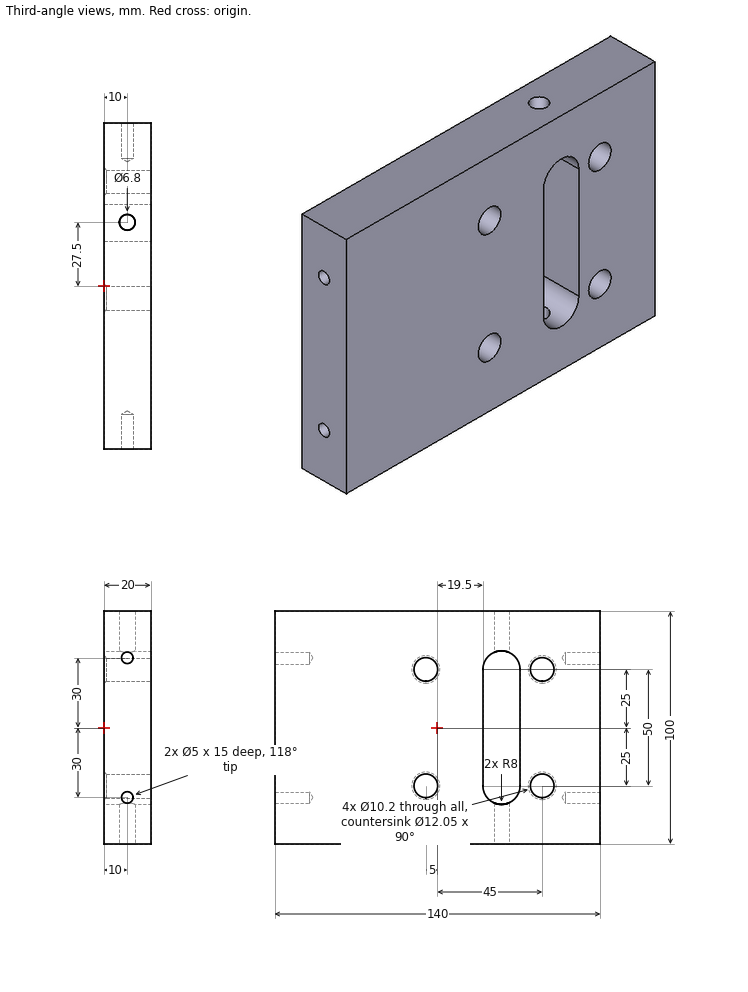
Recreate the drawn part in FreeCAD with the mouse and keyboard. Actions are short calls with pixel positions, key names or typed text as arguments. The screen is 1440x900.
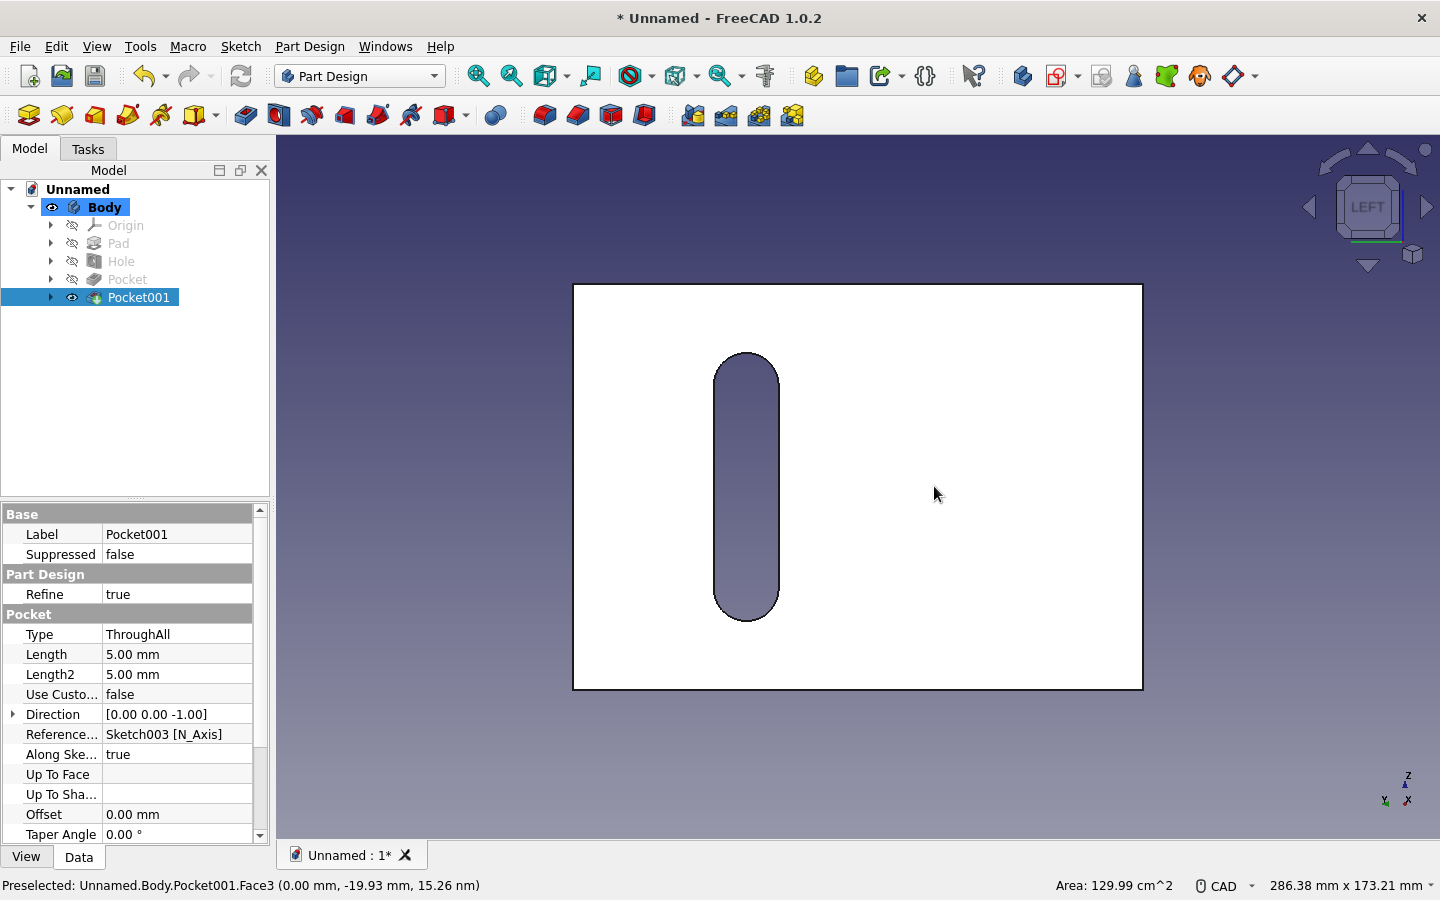
click(1056, 76)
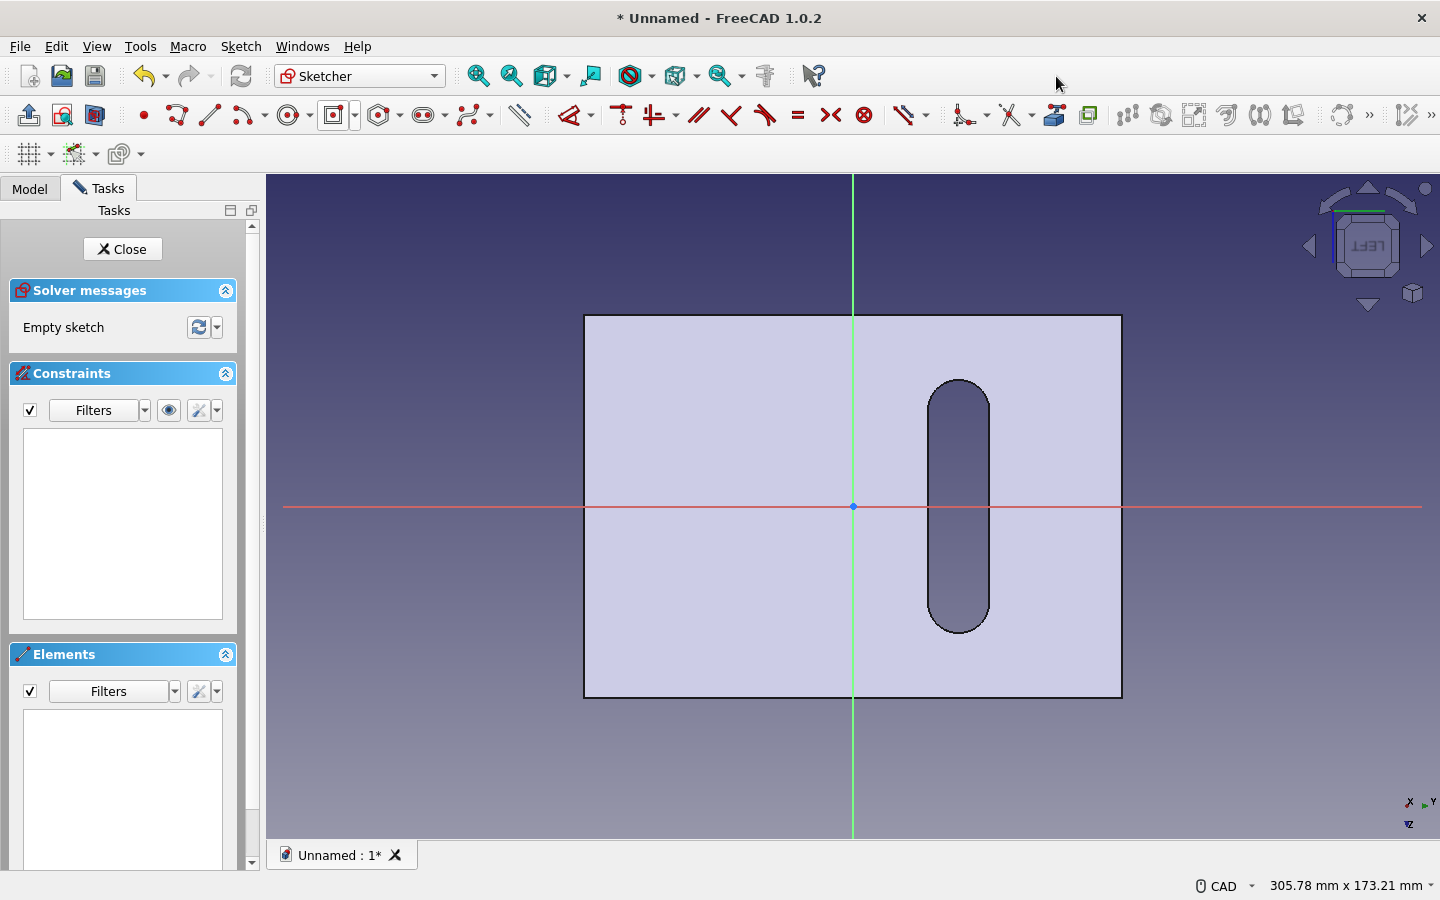
scroll(1107, 506, up, 3)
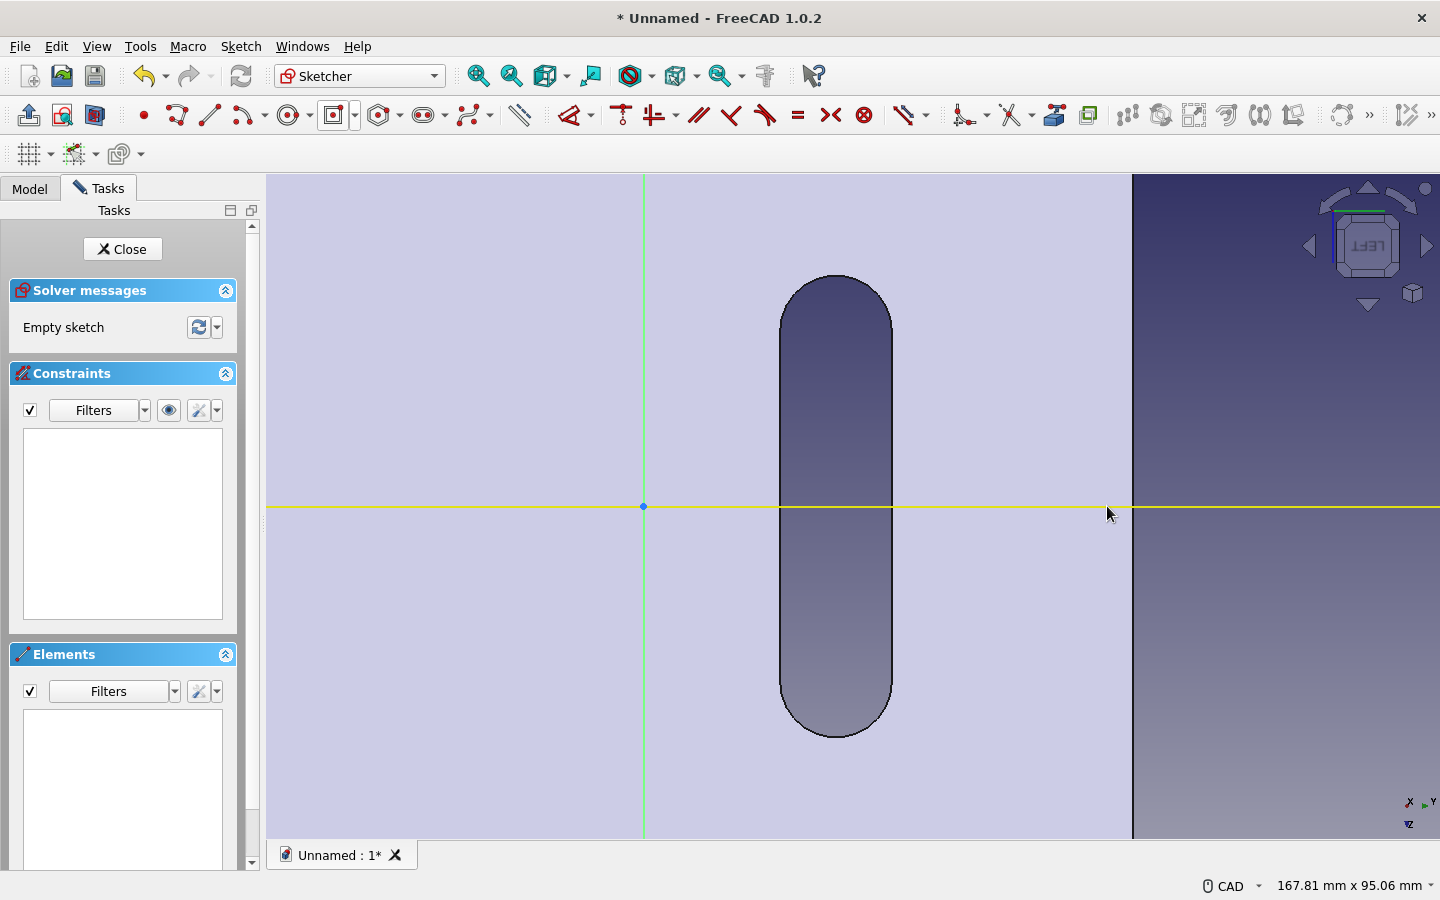
click(288, 116)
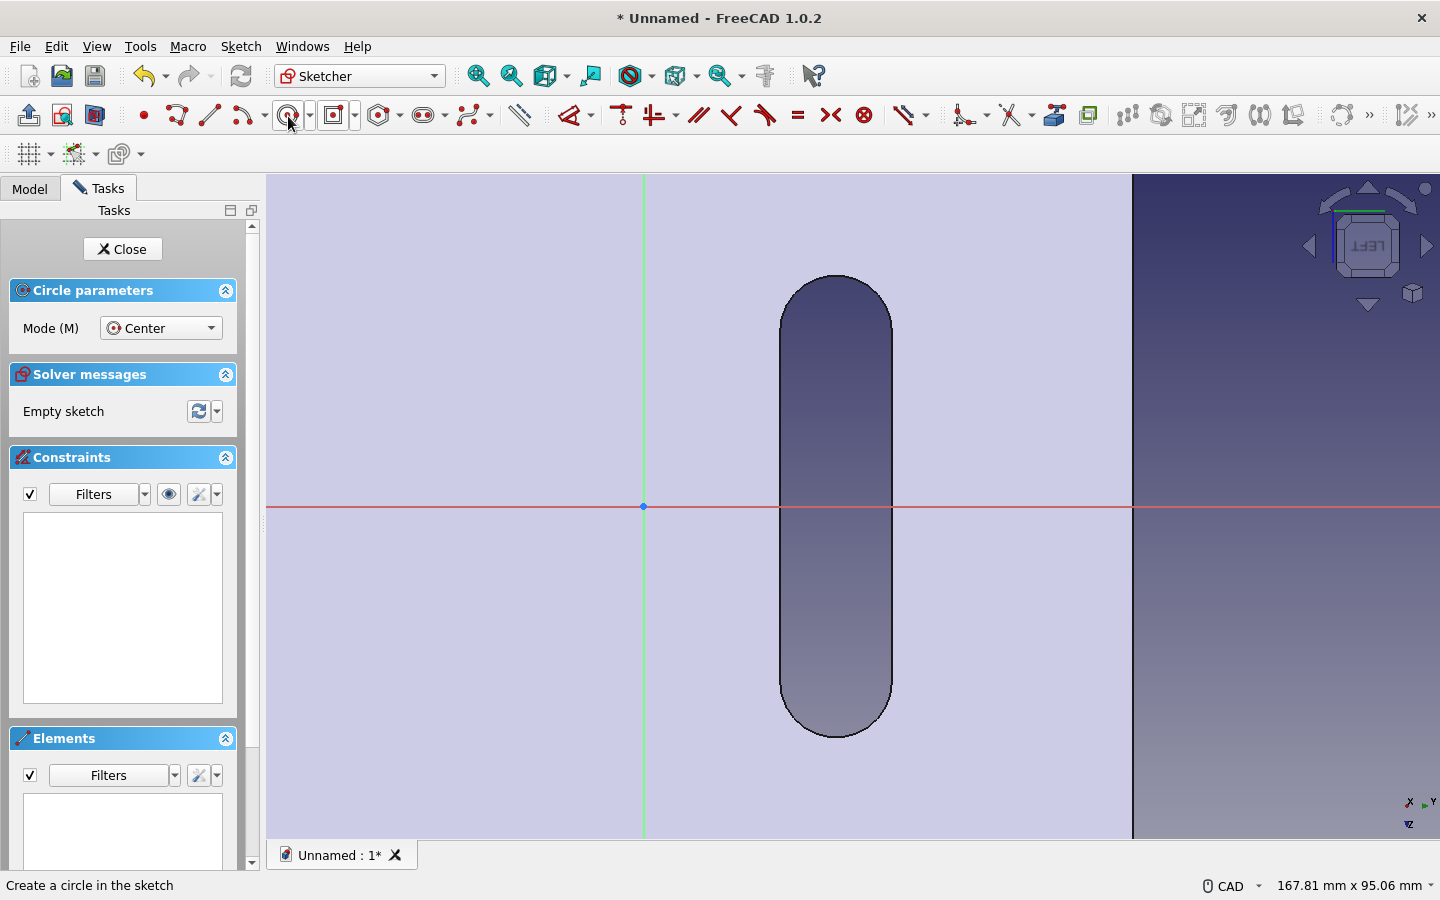
click(958, 332)
move(984, 306)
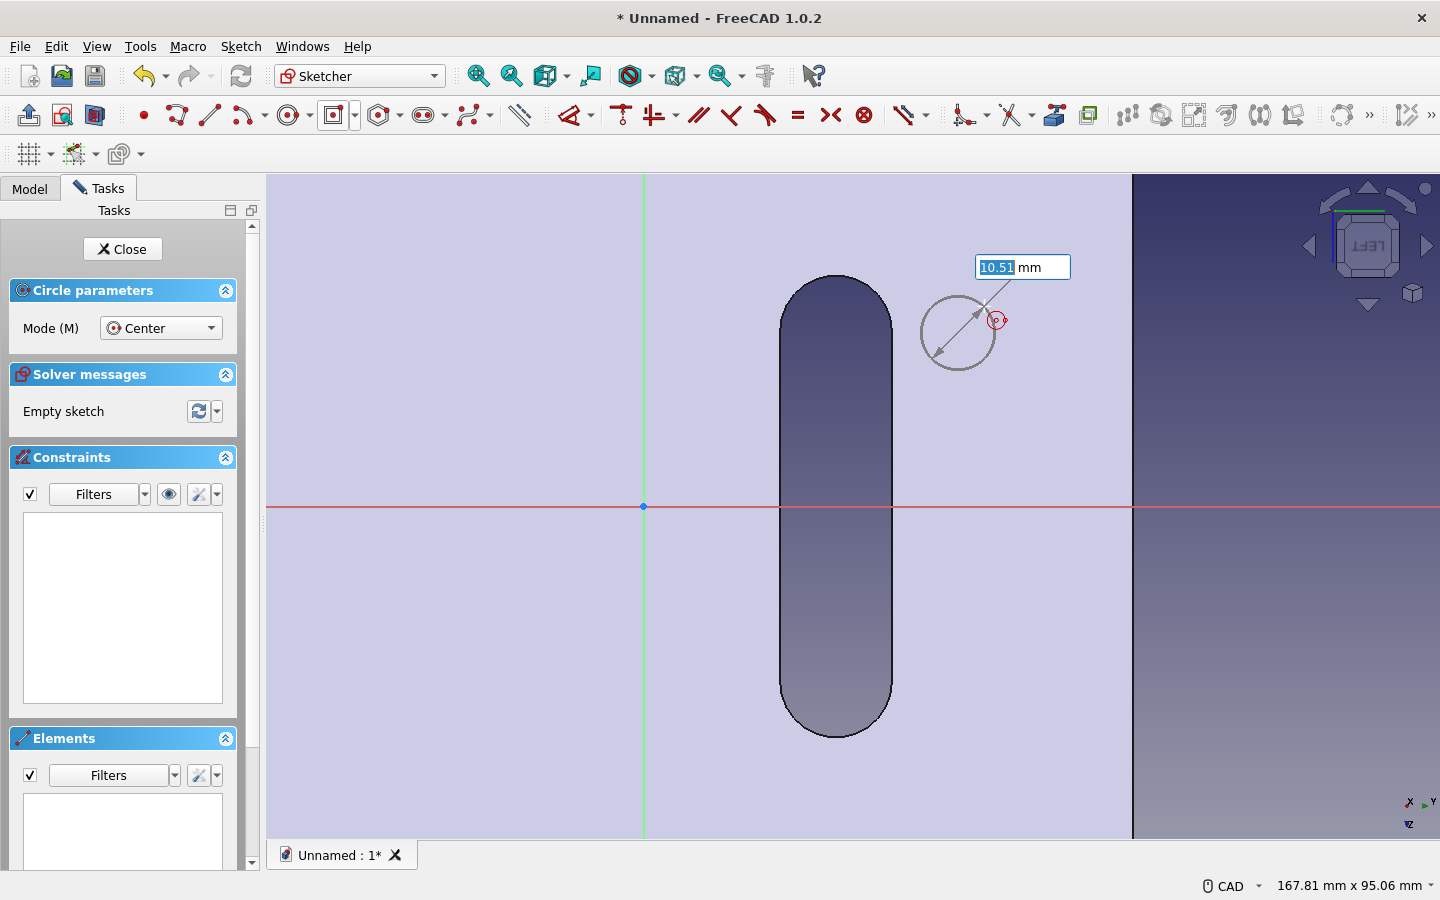
text(10.2)
key(Return)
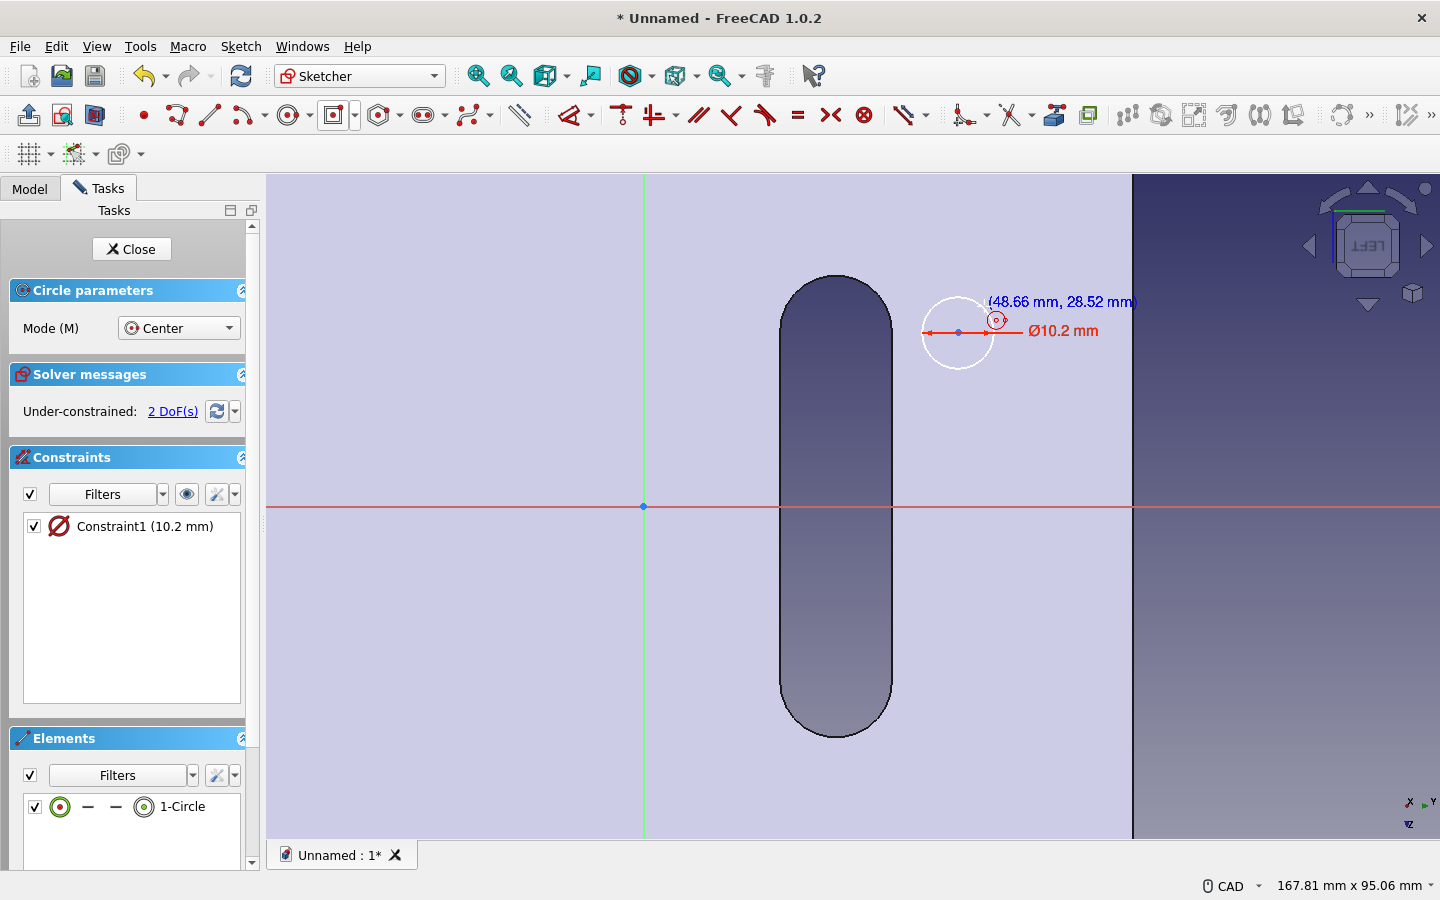
click(958, 681)
move(984, 656)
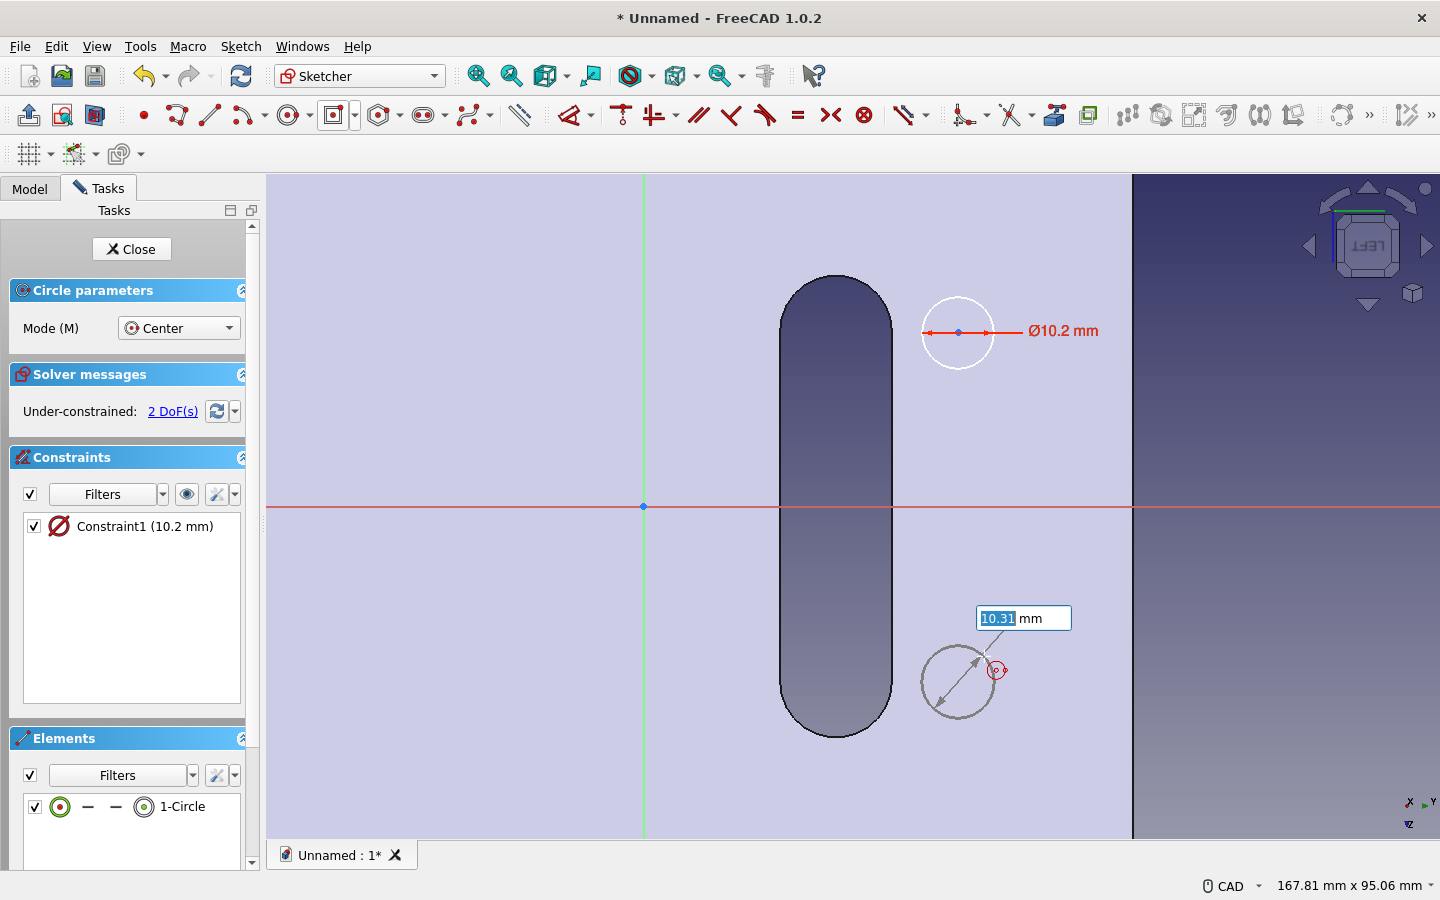
text(10.2)
key(Return)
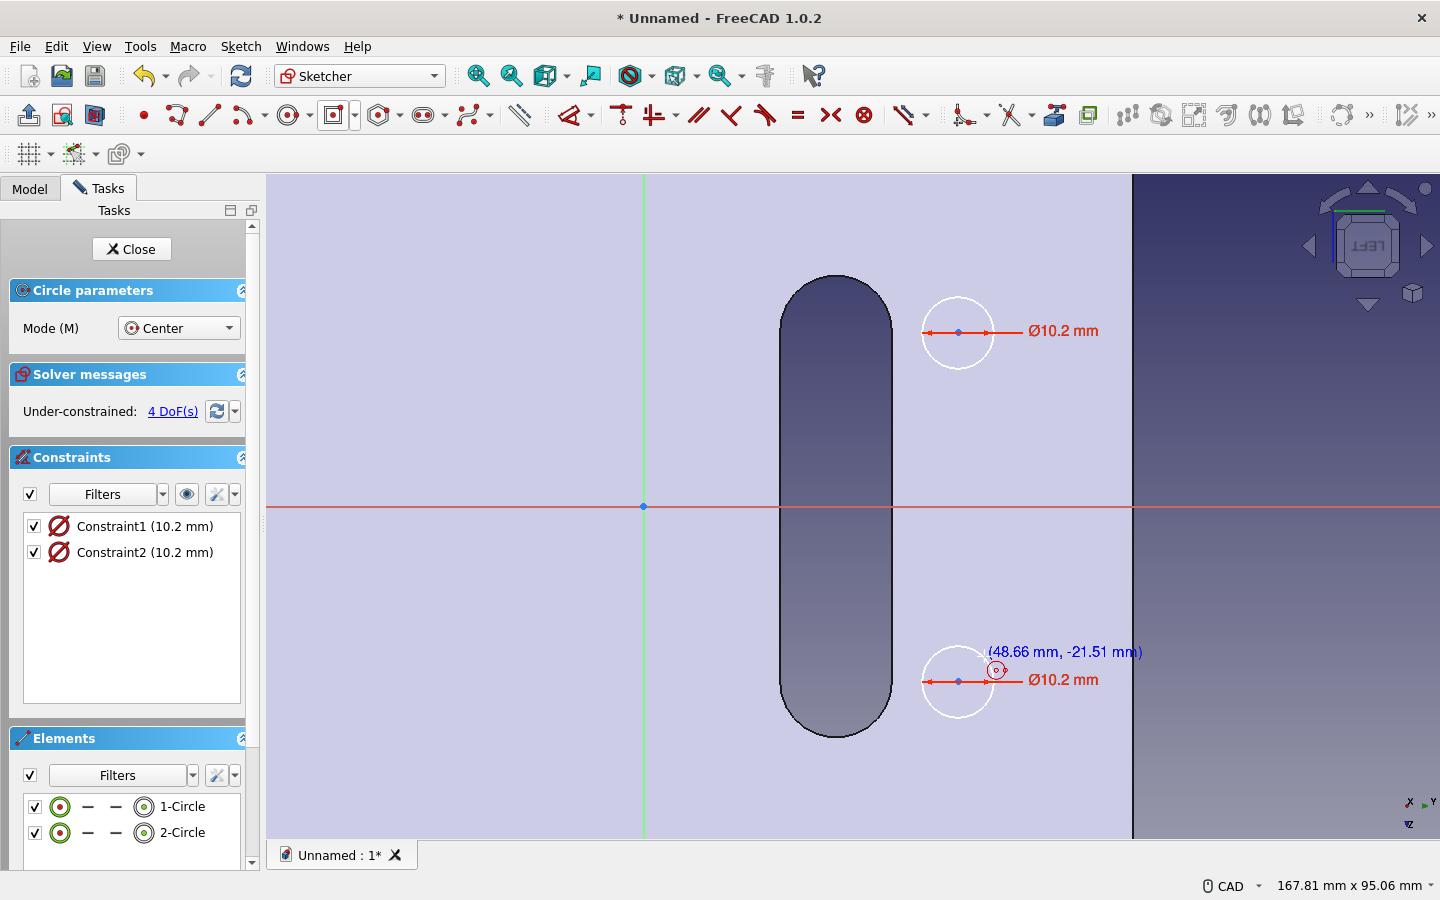
click(609, 332)
move(583, 306)